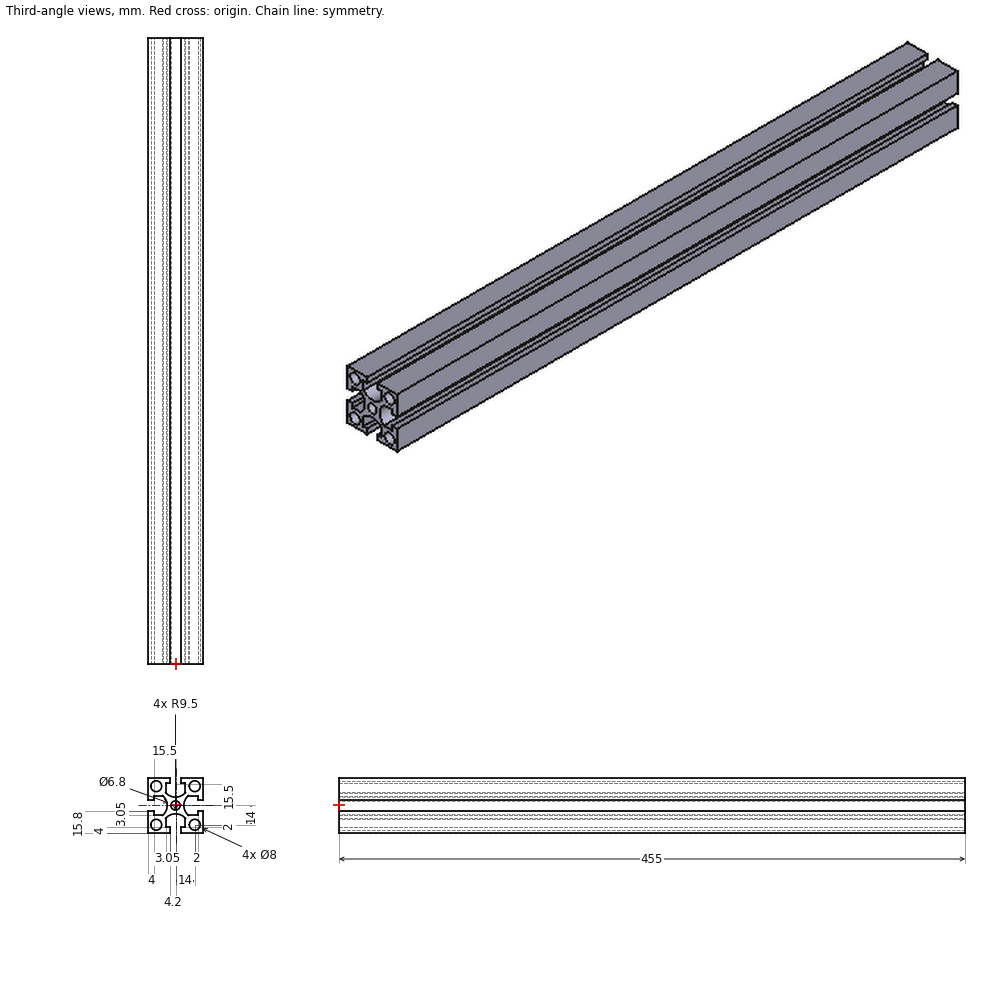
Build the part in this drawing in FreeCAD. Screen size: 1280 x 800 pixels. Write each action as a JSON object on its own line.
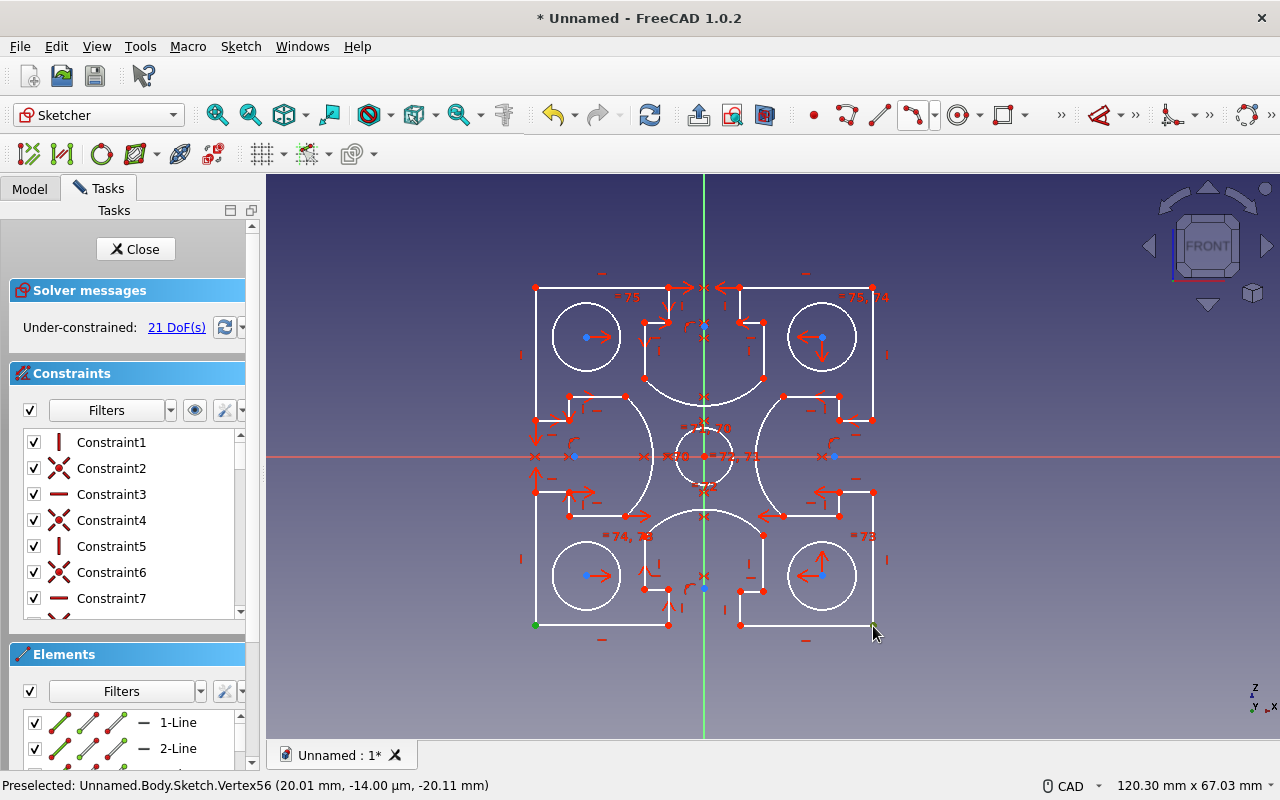
{"action": "left_click", "coordinate": [704, 675]}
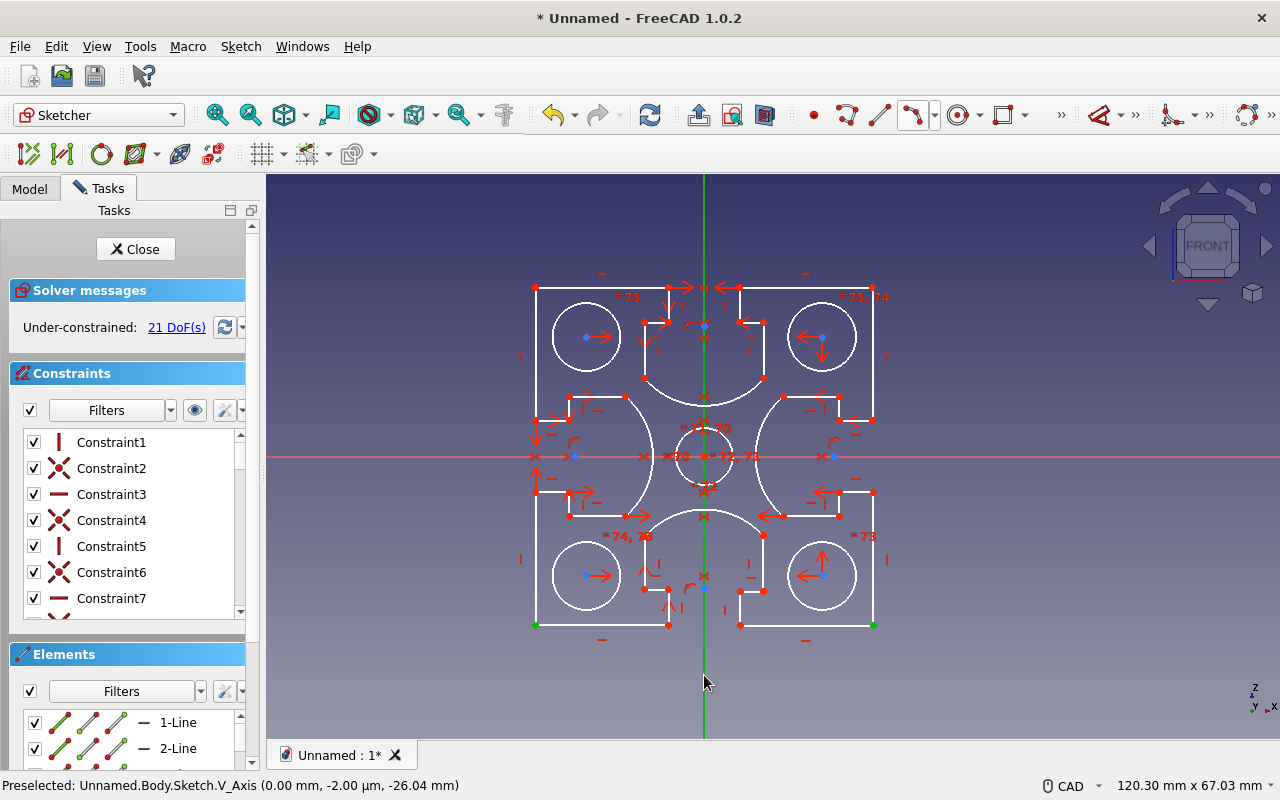
{"action": "key", "text": "s"}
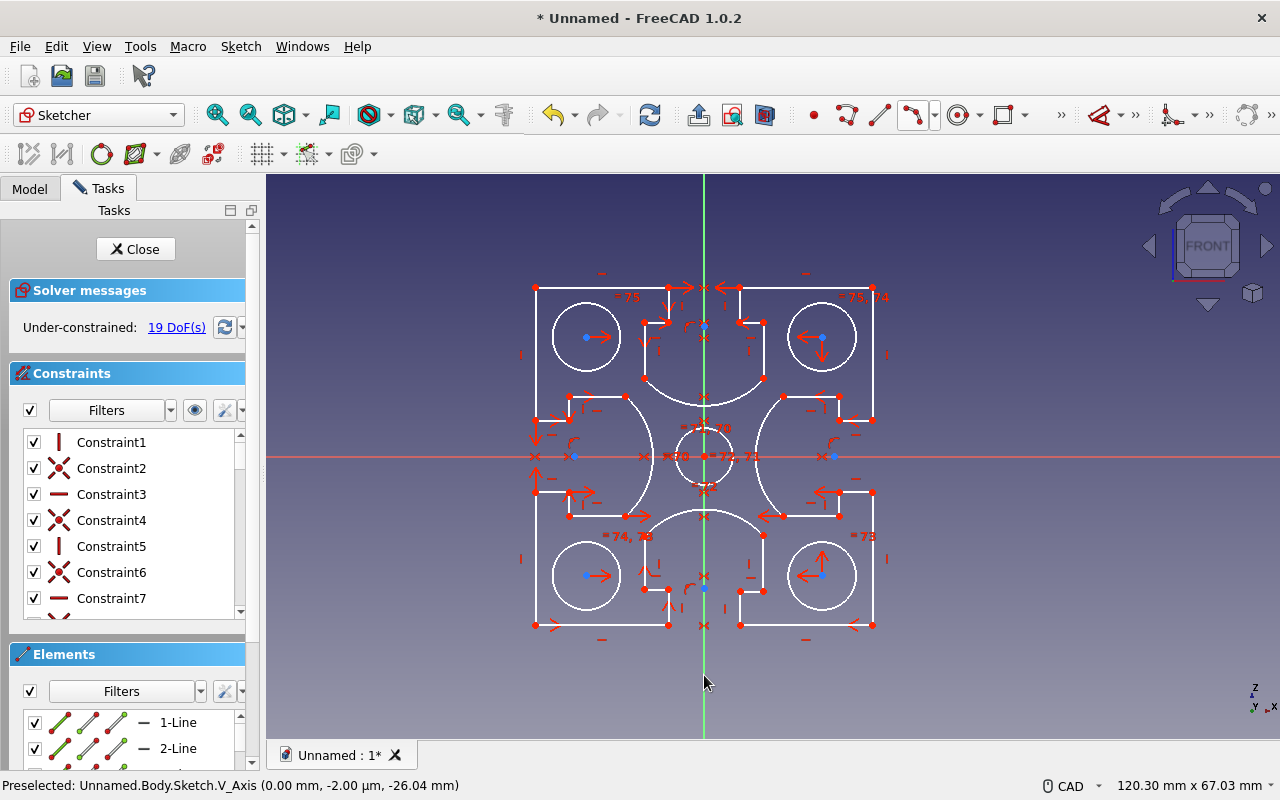
{"action": "left_click", "coordinate": [669, 590]}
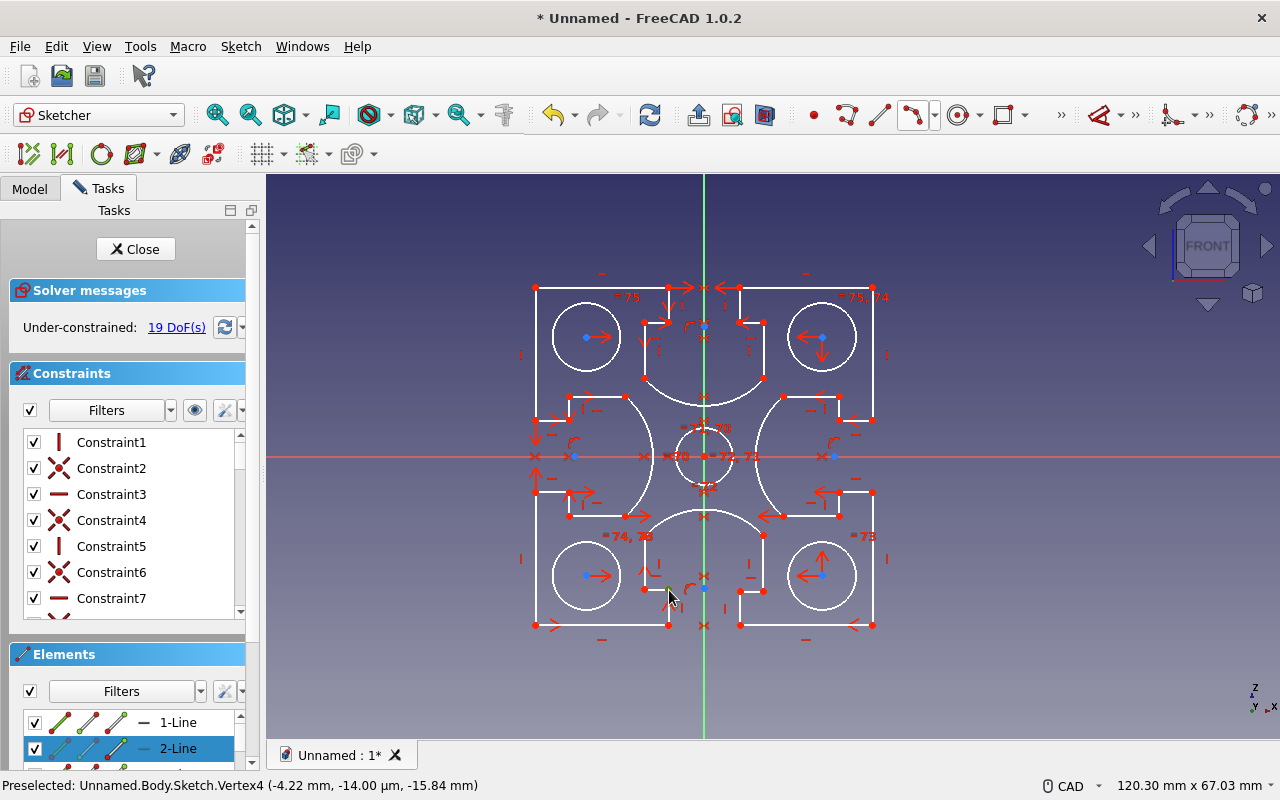
{"action": "left_click", "coordinate": [740, 592]}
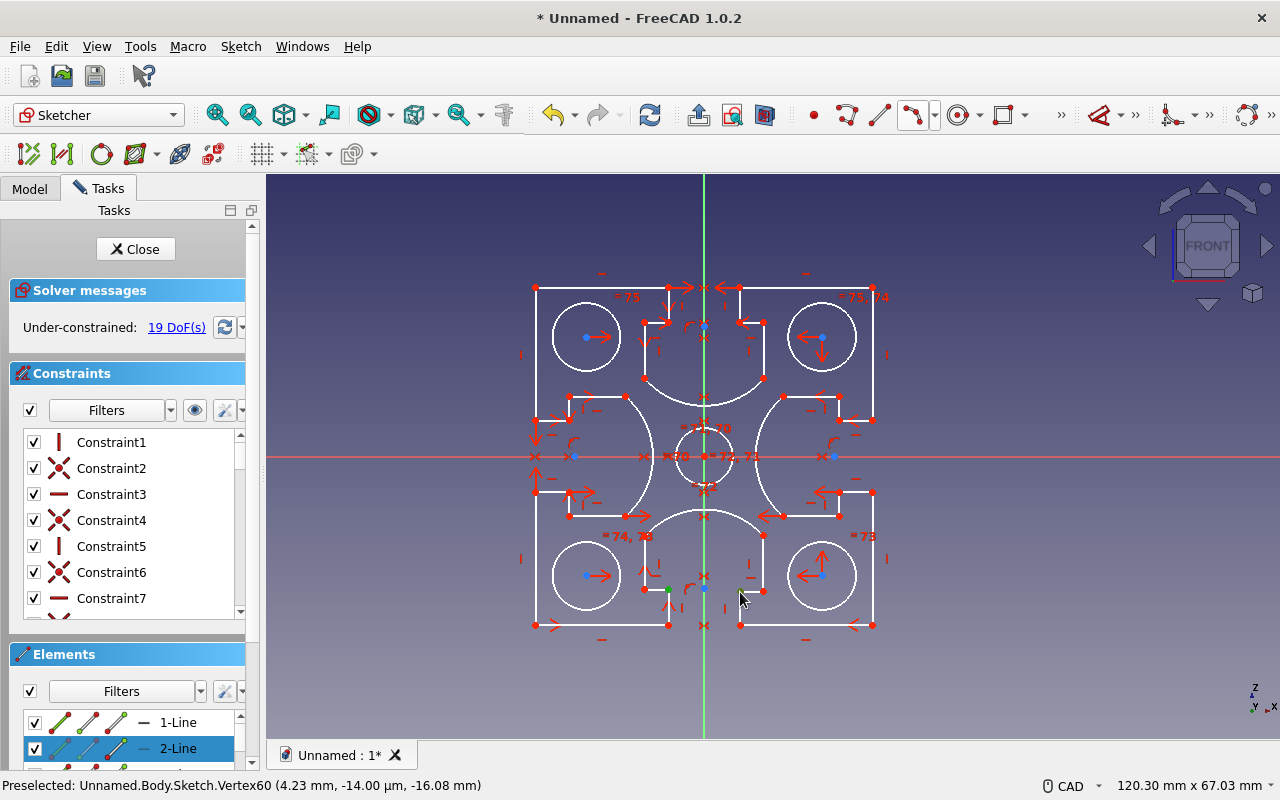
{"action": "left_click", "coordinate": [704, 675]}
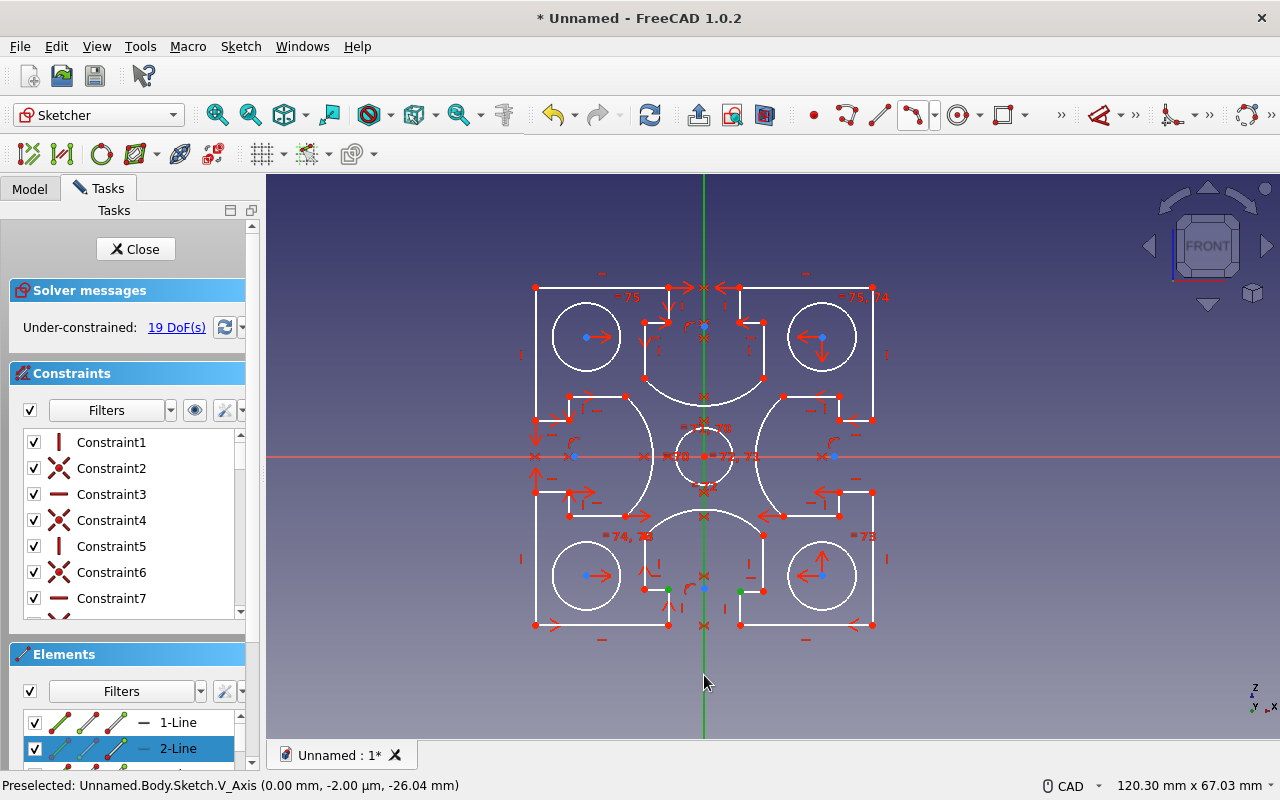
{"action": "key", "text": "s"}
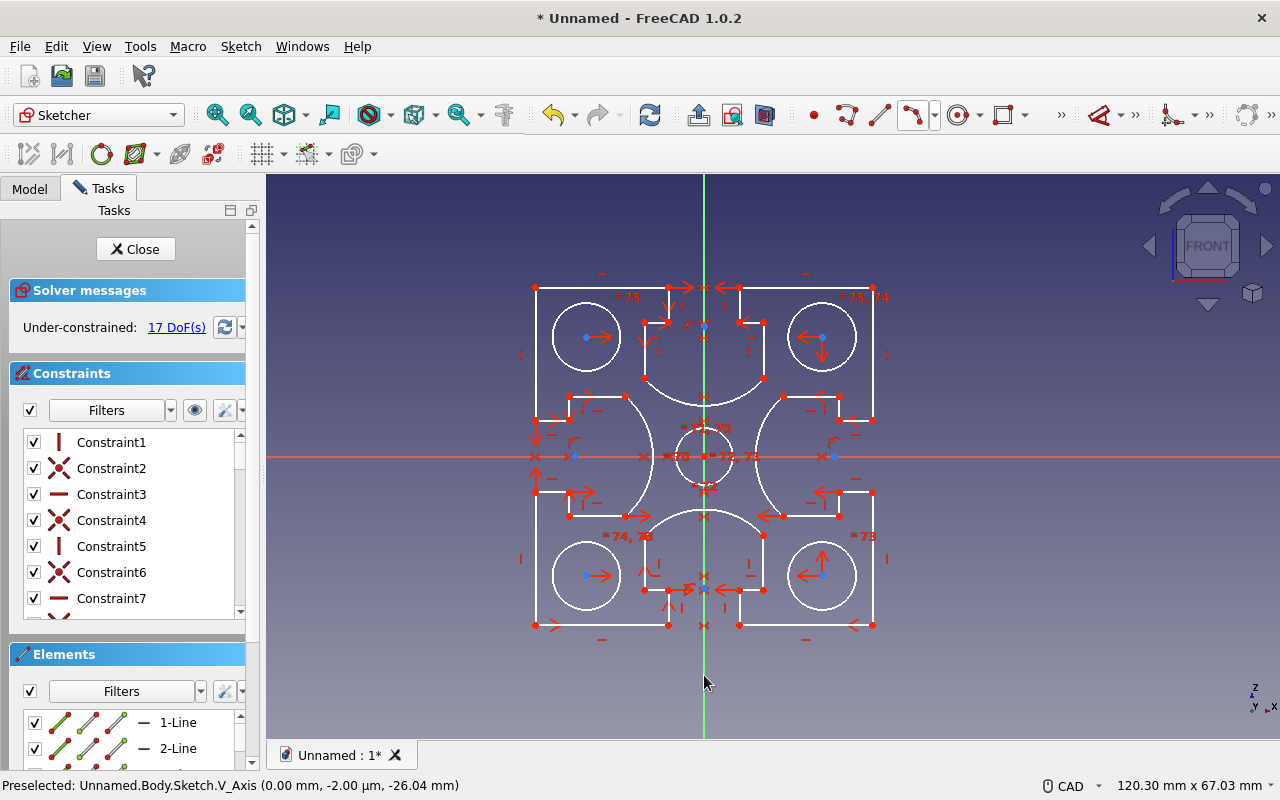
{"action": "left_click", "coordinate": [764, 379]}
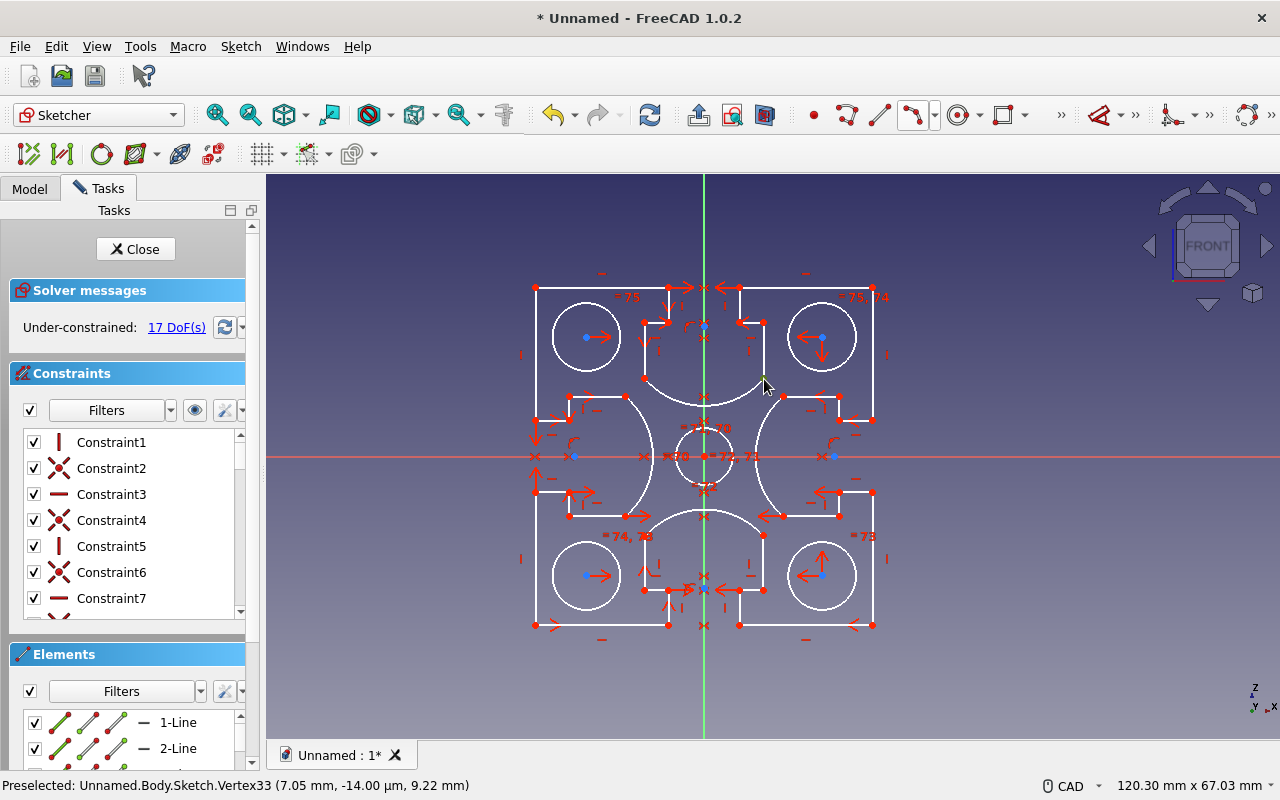
{"action": "left_click", "coordinate": [763, 536]}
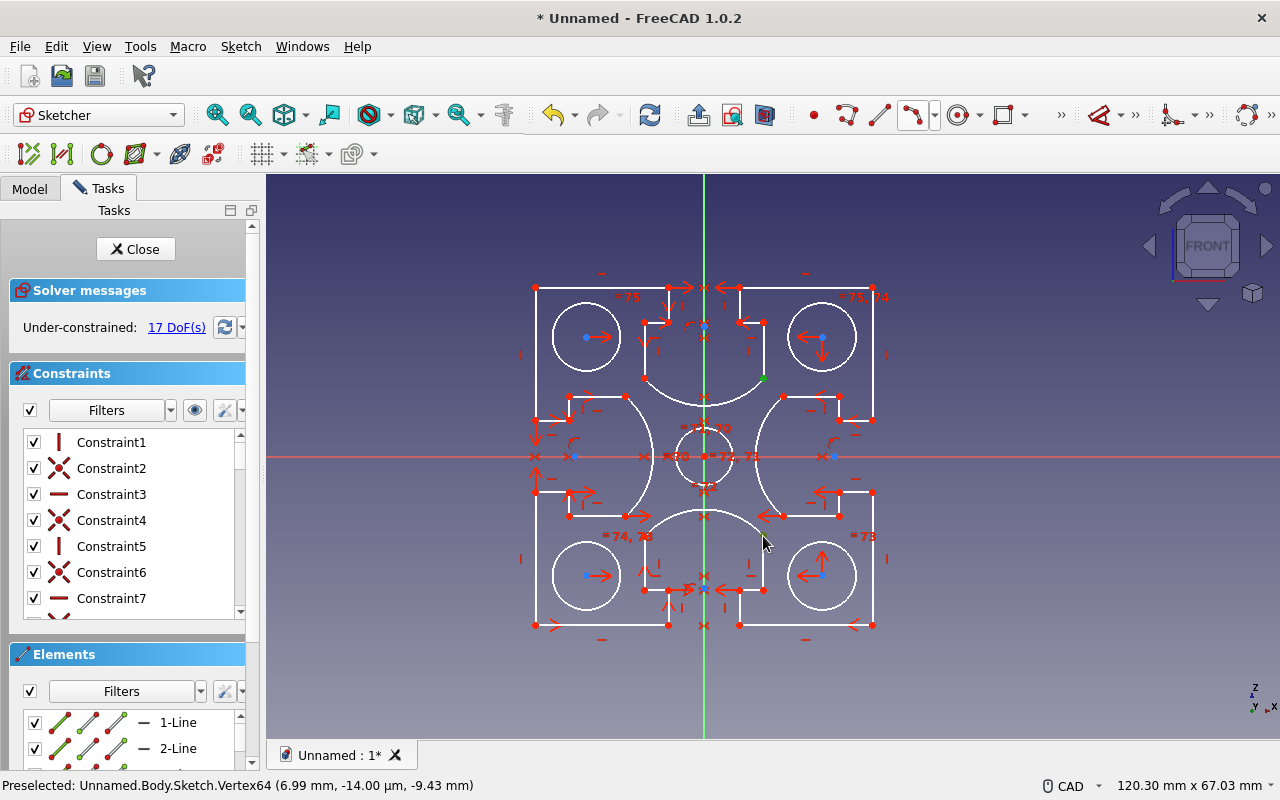
{"action": "left_click", "coordinate": [353, 456]}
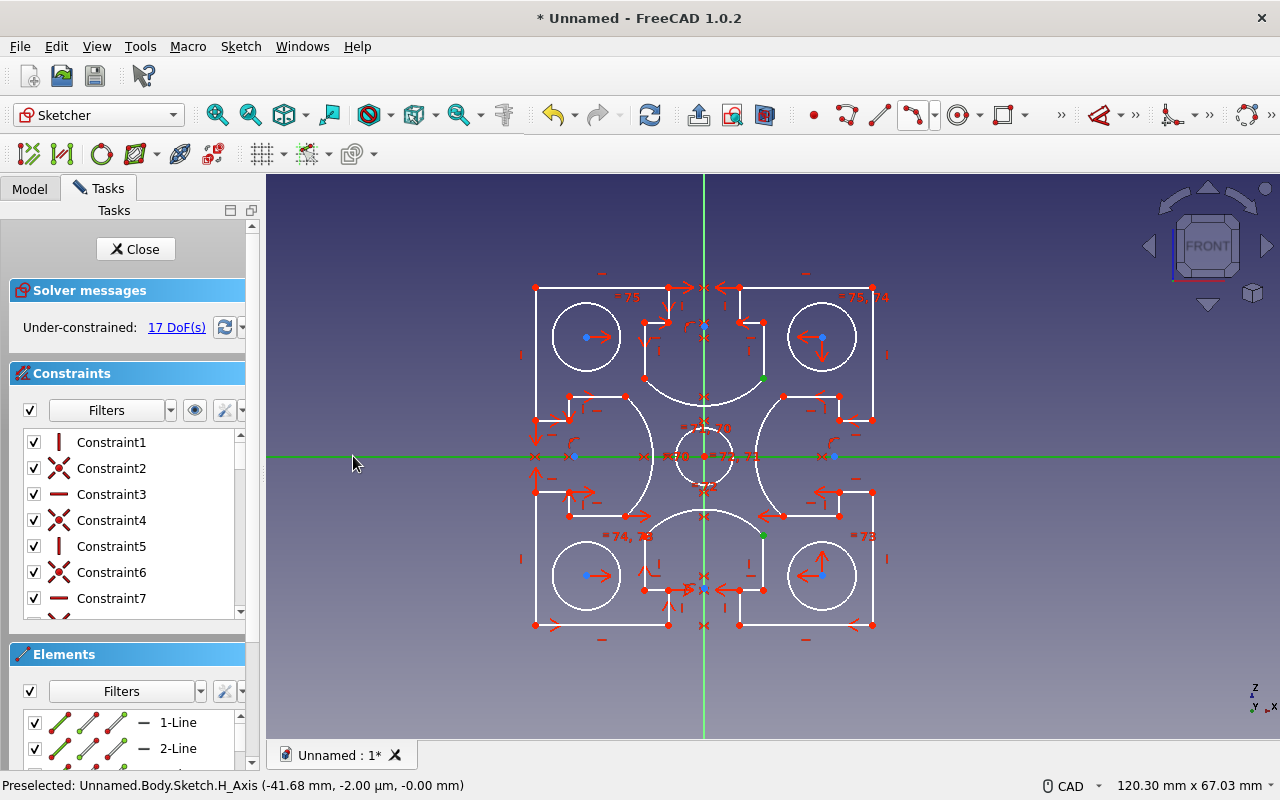
{"action": "key", "text": "s"}